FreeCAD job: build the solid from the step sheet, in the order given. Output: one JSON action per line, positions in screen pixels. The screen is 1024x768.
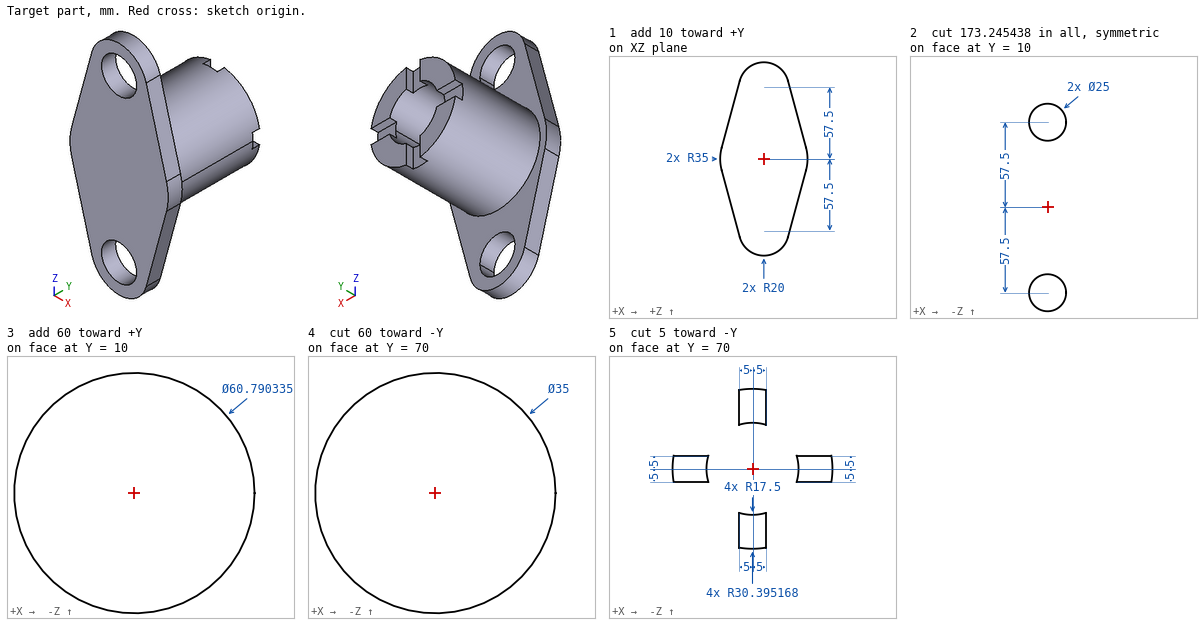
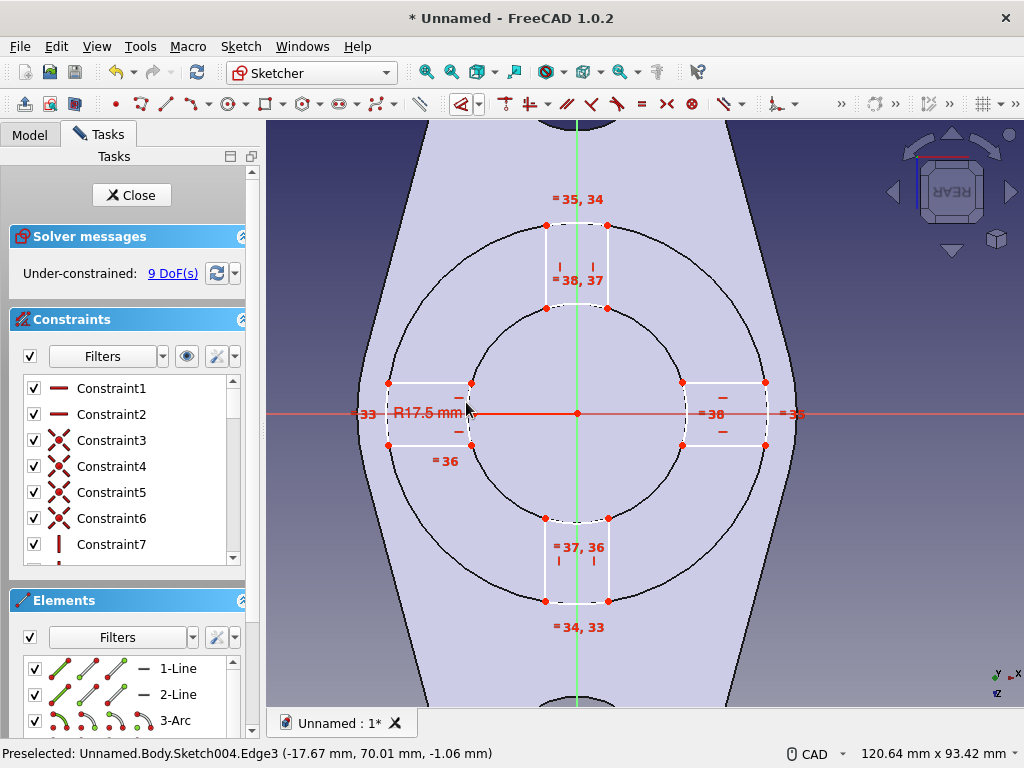
{"action": "left_click", "coordinate": [387, 402]}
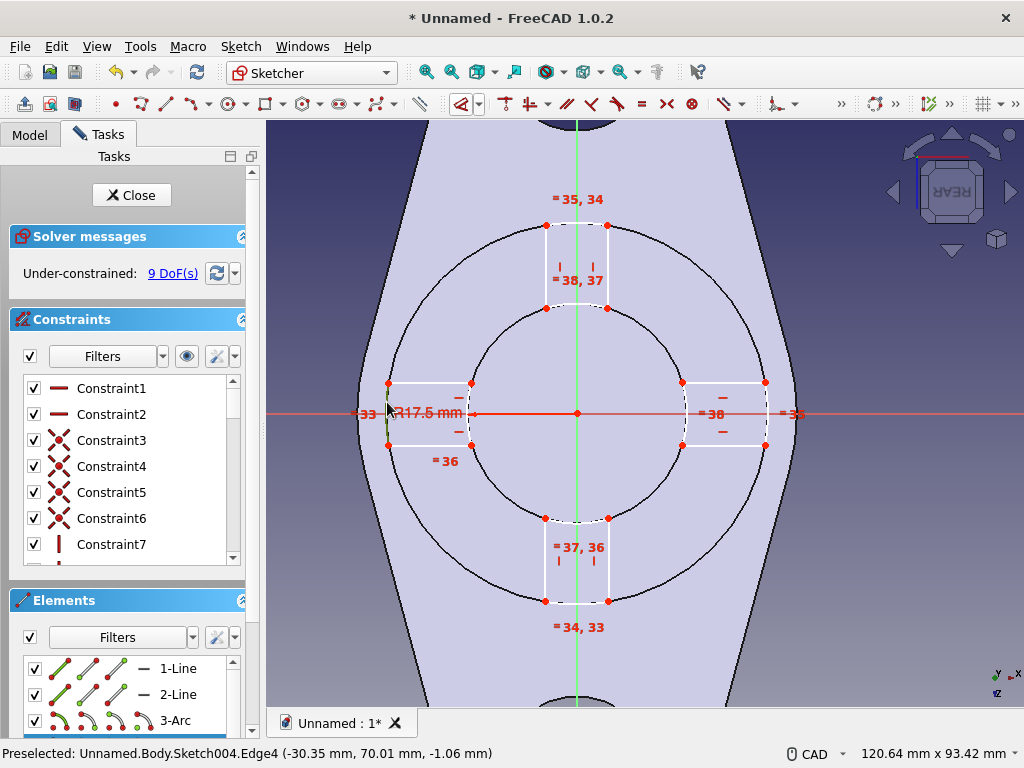
{"action": "left_click", "coordinate": [478, 104]}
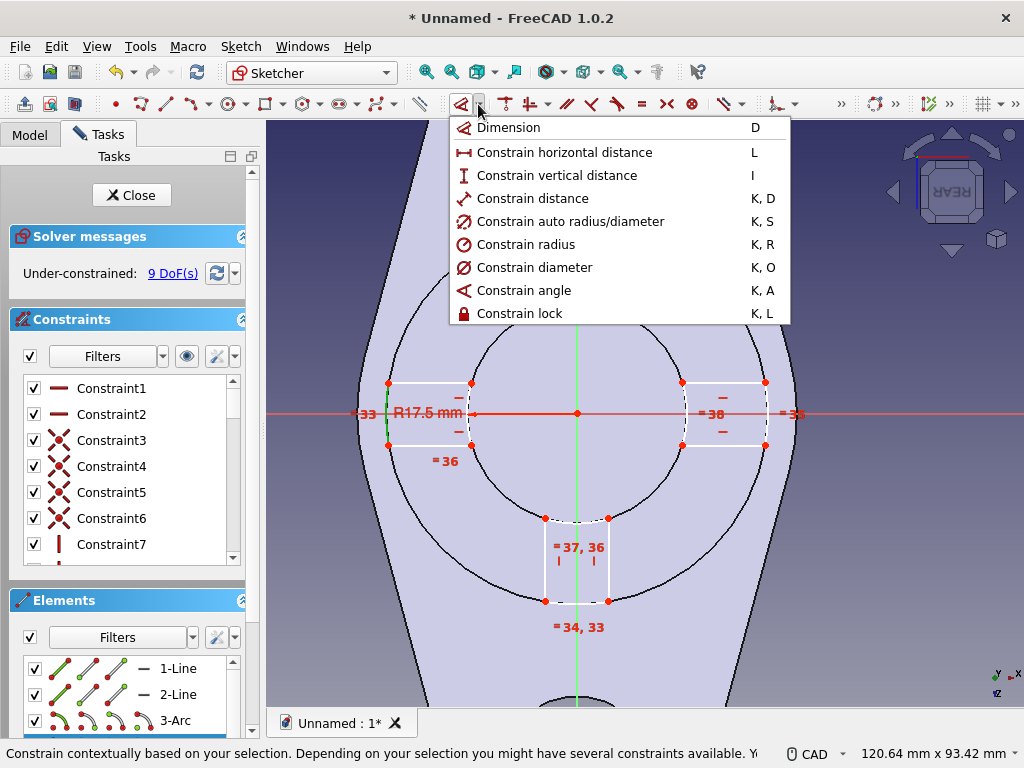
{"action": "left_click", "coordinate": [620, 244]}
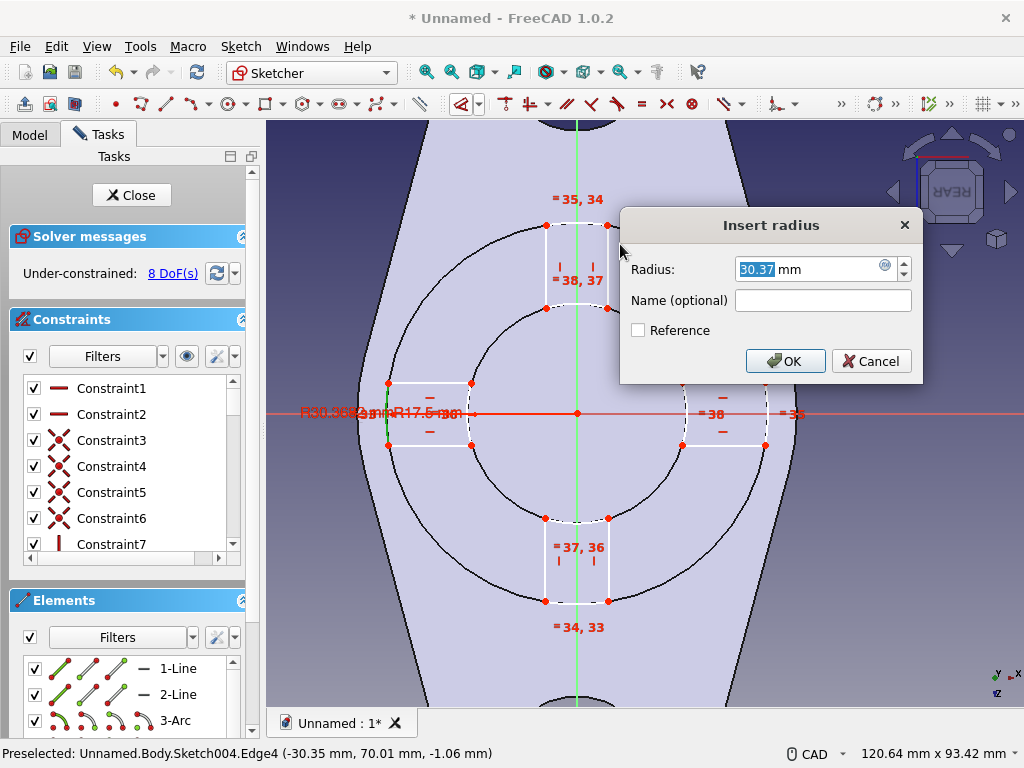
{"action": "type", "text": "30.395168"}
{"action": "key", "text": "Return"}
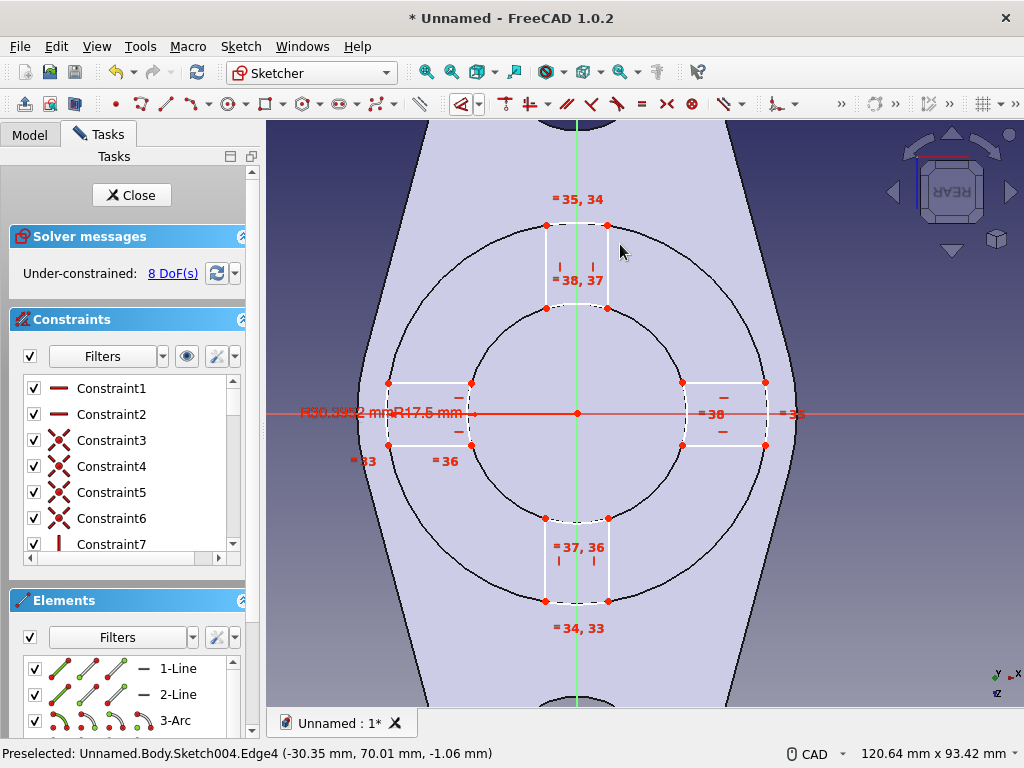
{"action": "scroll", "coordinate": [389, 446], "scroll_direction": "up", "scroll_amount": 2}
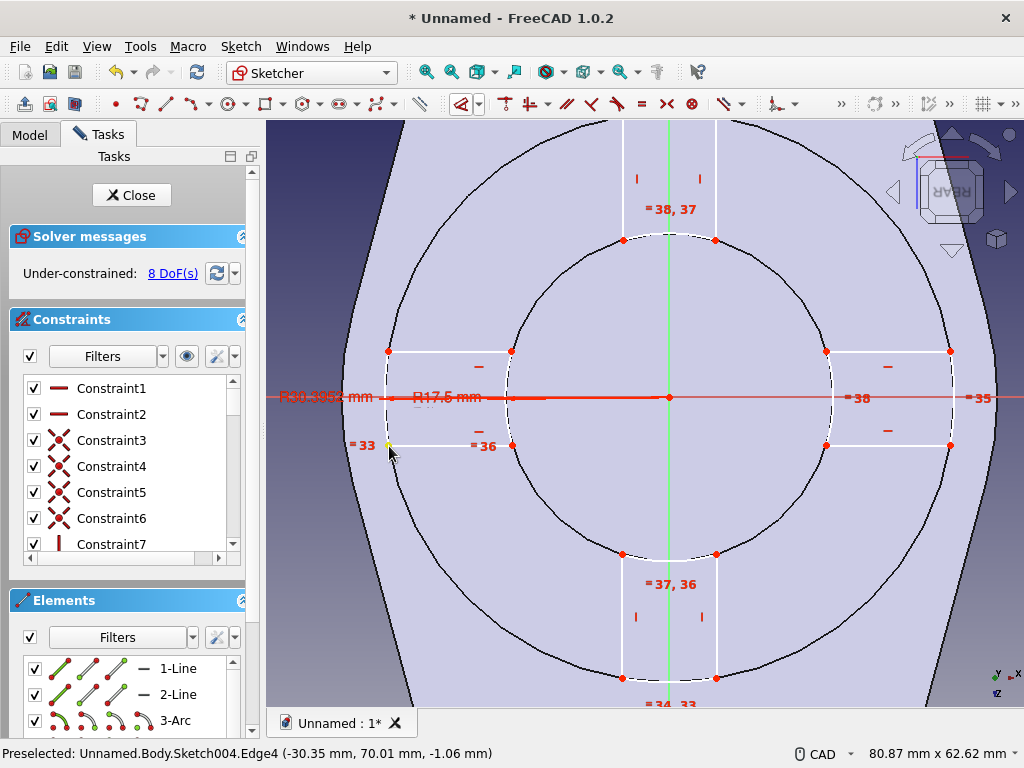
{"action": "left_click", "coordinate": [389, 446]}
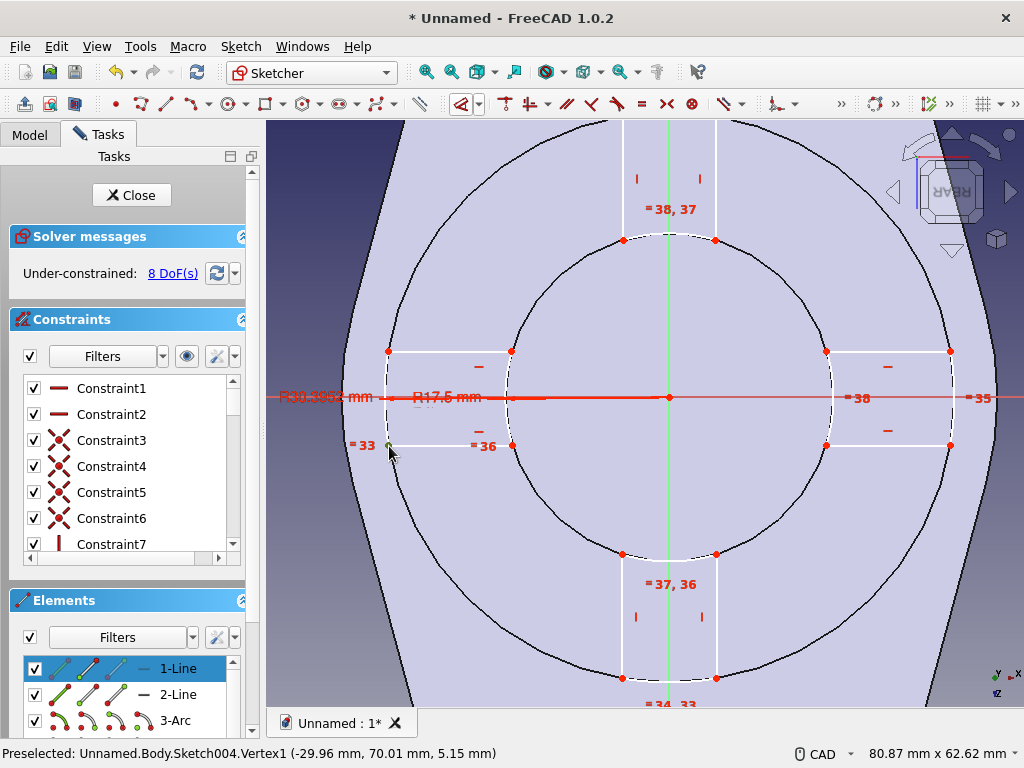
{"action": "key", "text": "i"}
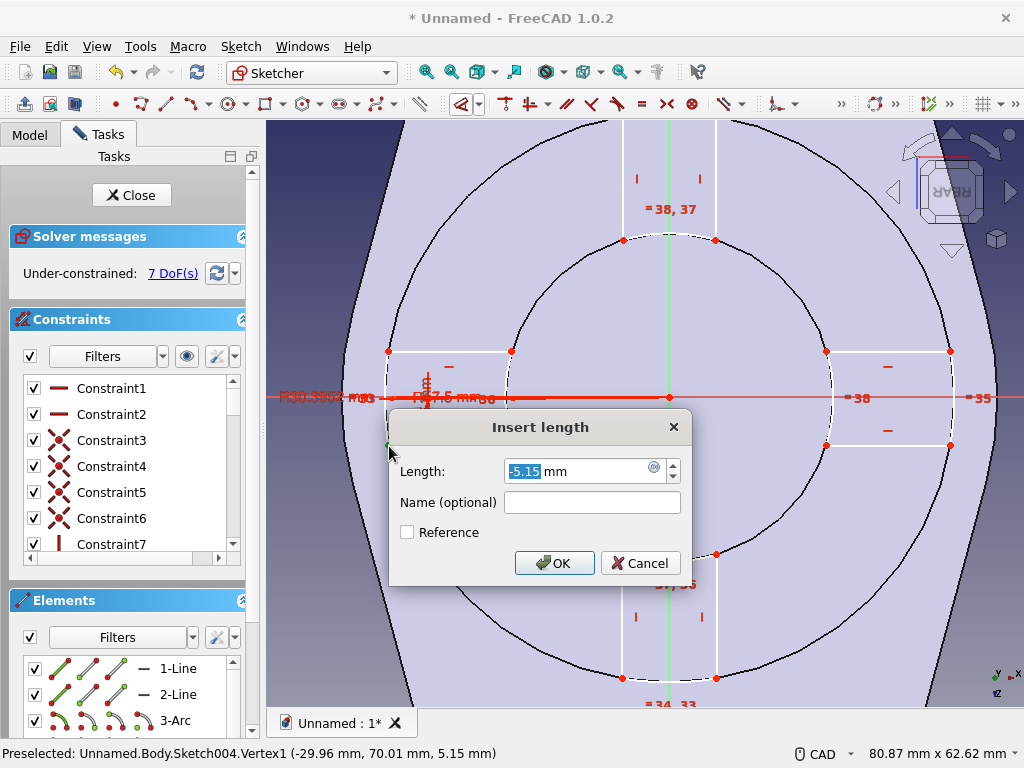
{"action": "type", "text": "-5"}
{"action": "key", "text": "Return"}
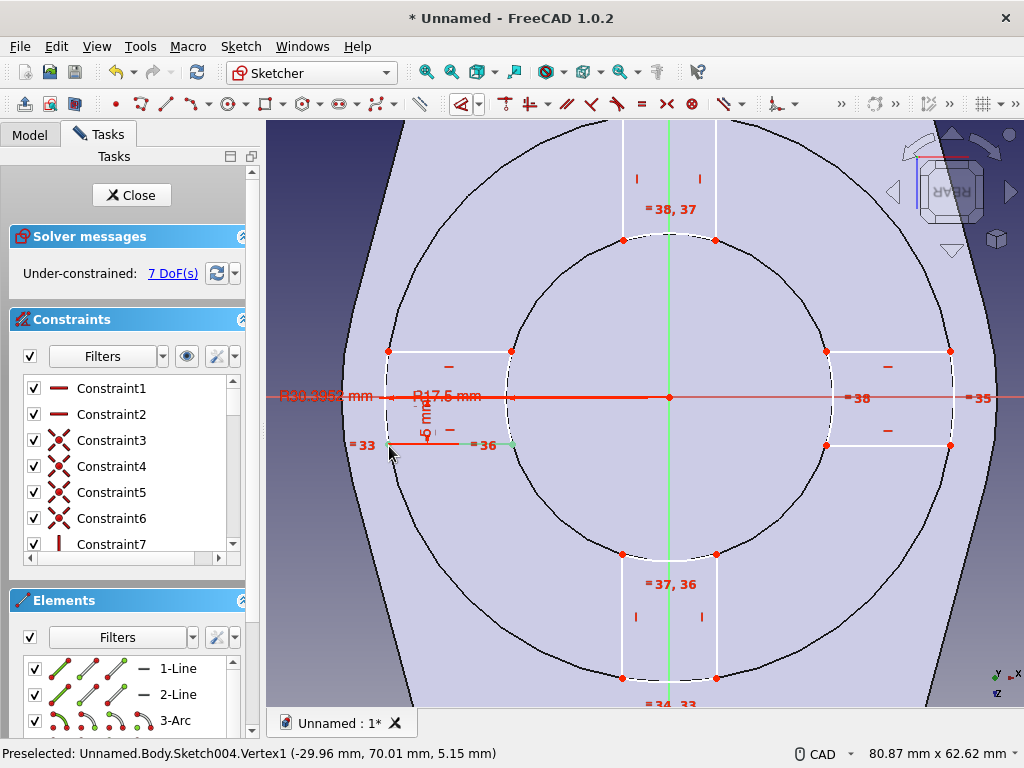
{"action": "left_click", "coordinate": [512, 352]}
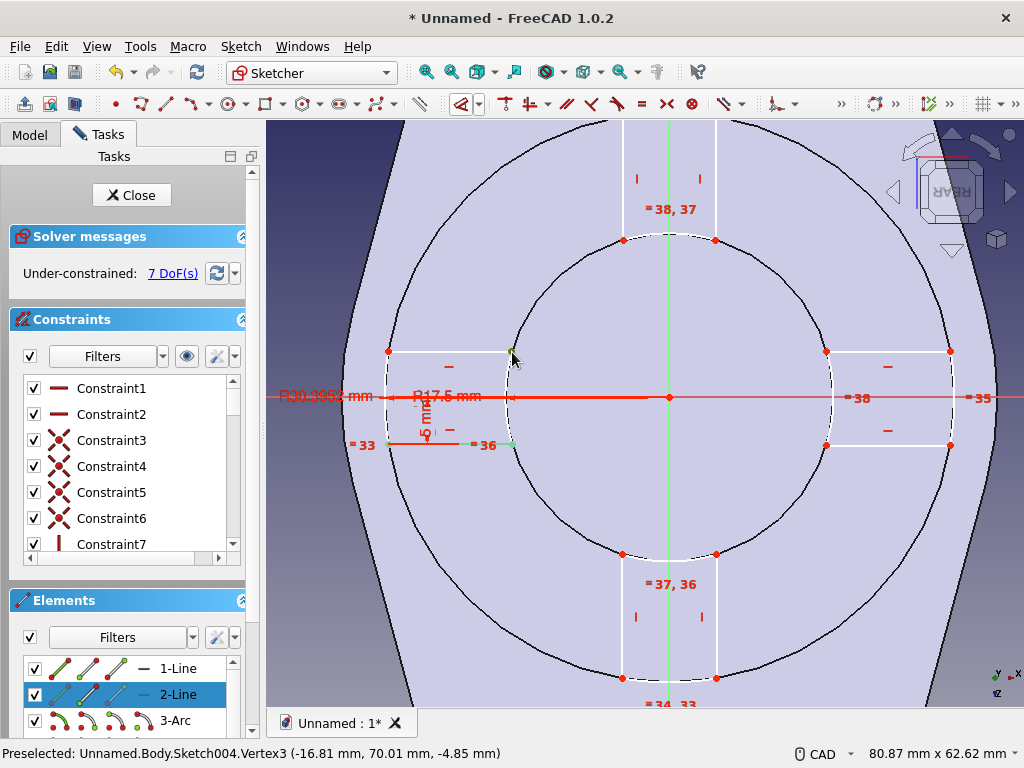
{"action": "key", "text": "i"}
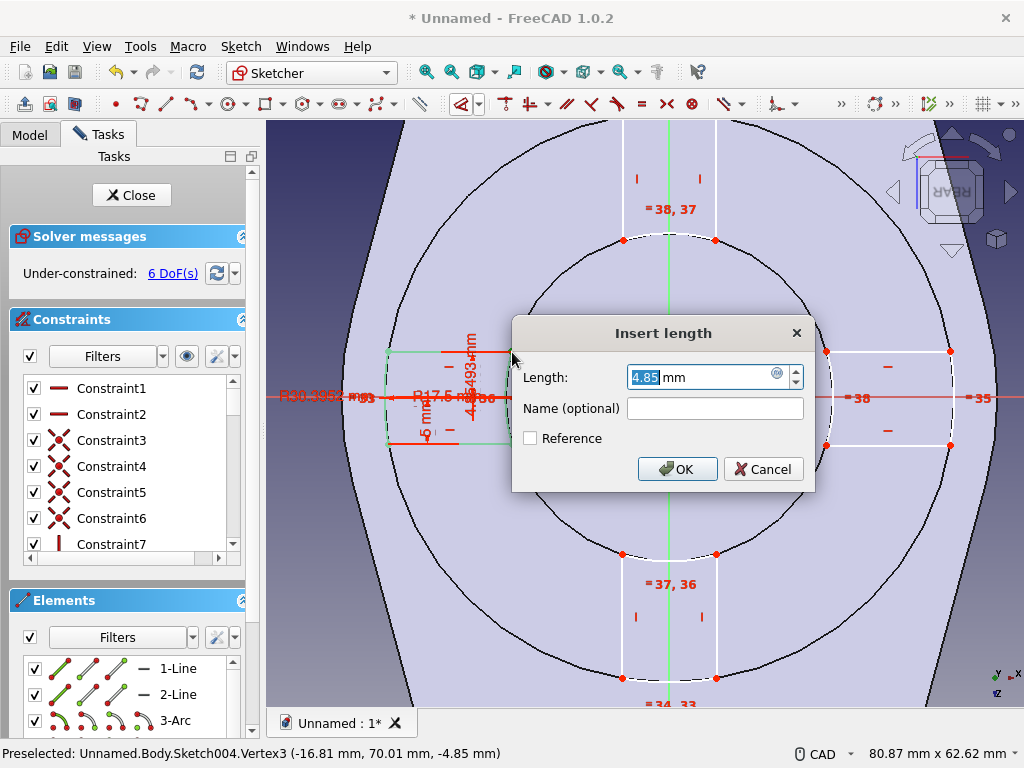
{"action": "type", "text": "5"}
{"action": "key", "text": "Return"}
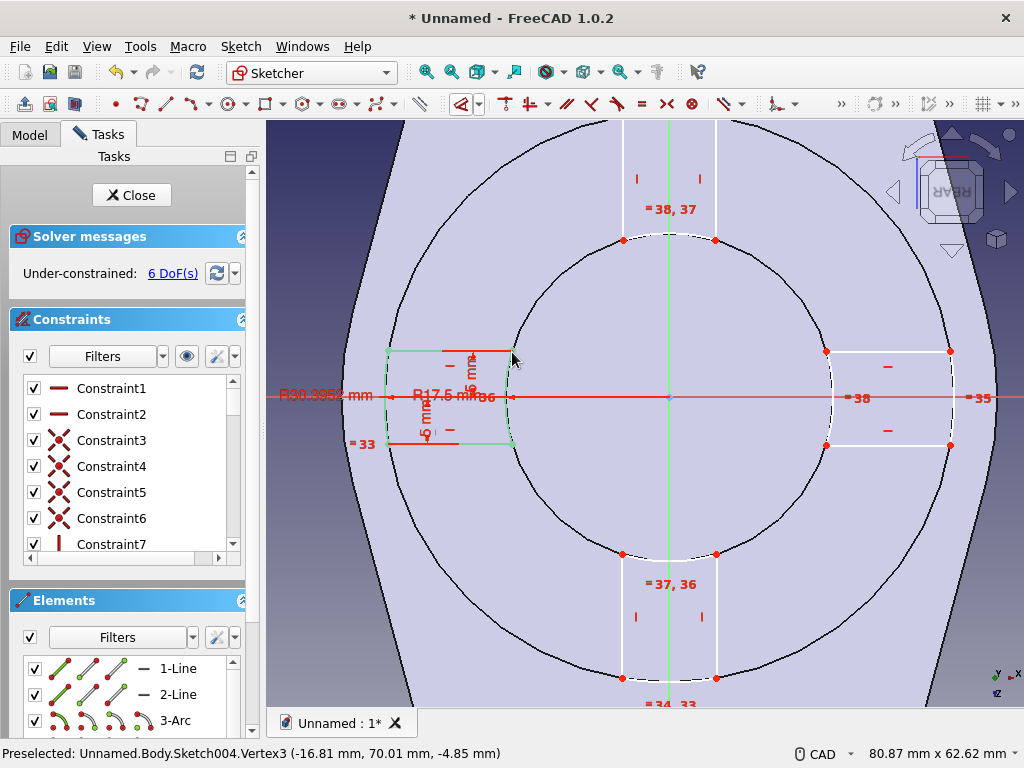
{"action": "left_click", "coordinate": [622, 554]}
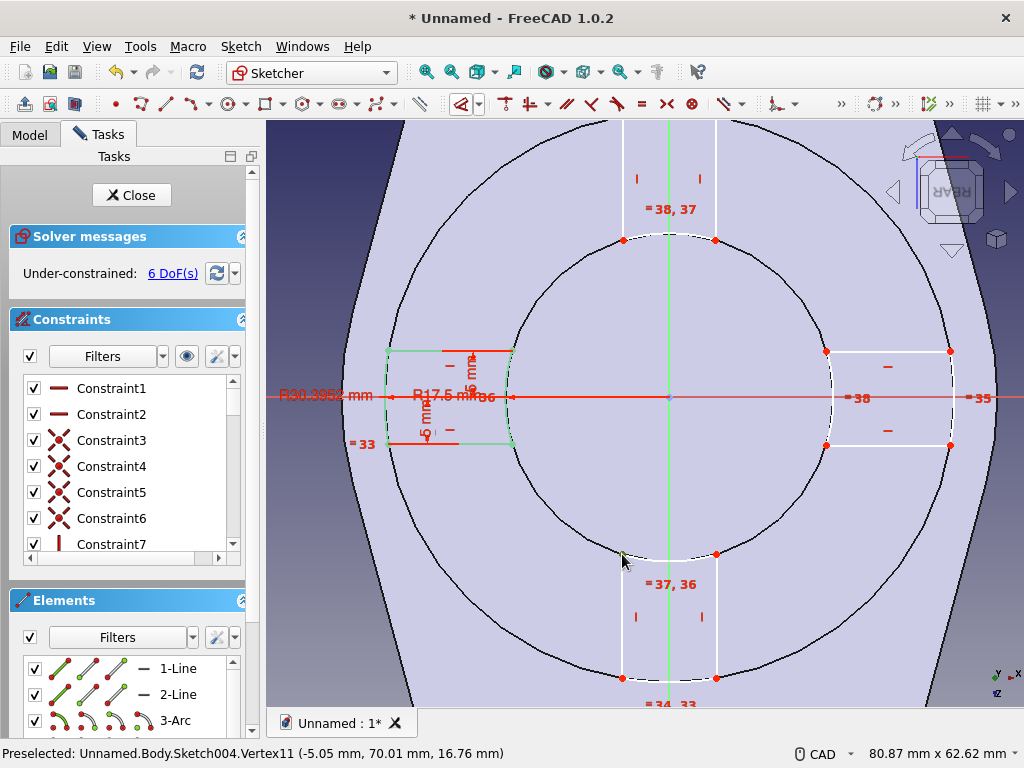
{"action": "key", "text": "l"}